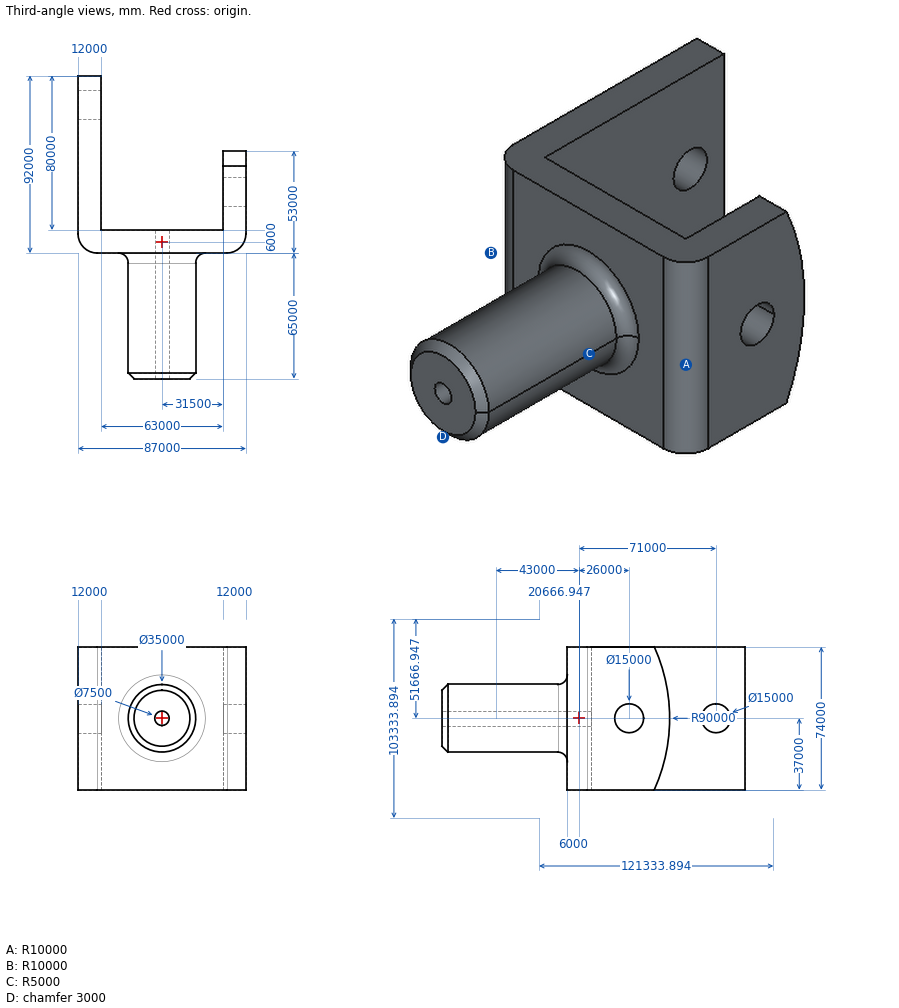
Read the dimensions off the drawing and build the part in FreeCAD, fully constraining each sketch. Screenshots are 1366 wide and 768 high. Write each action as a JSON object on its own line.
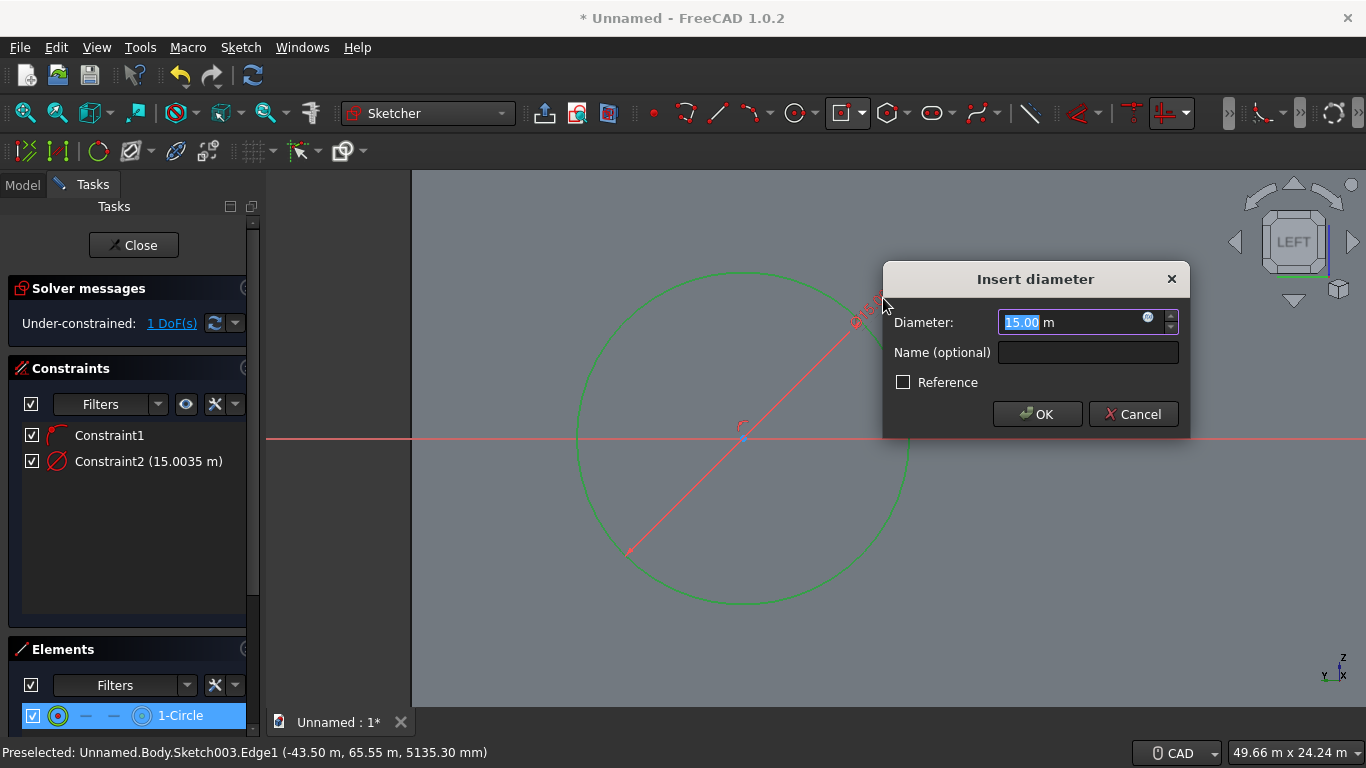
{"action": "key", "text": "ctrl+a"}
{"action": "type", "text": "15000 mm"}
{"action": "key", "text": "Return"}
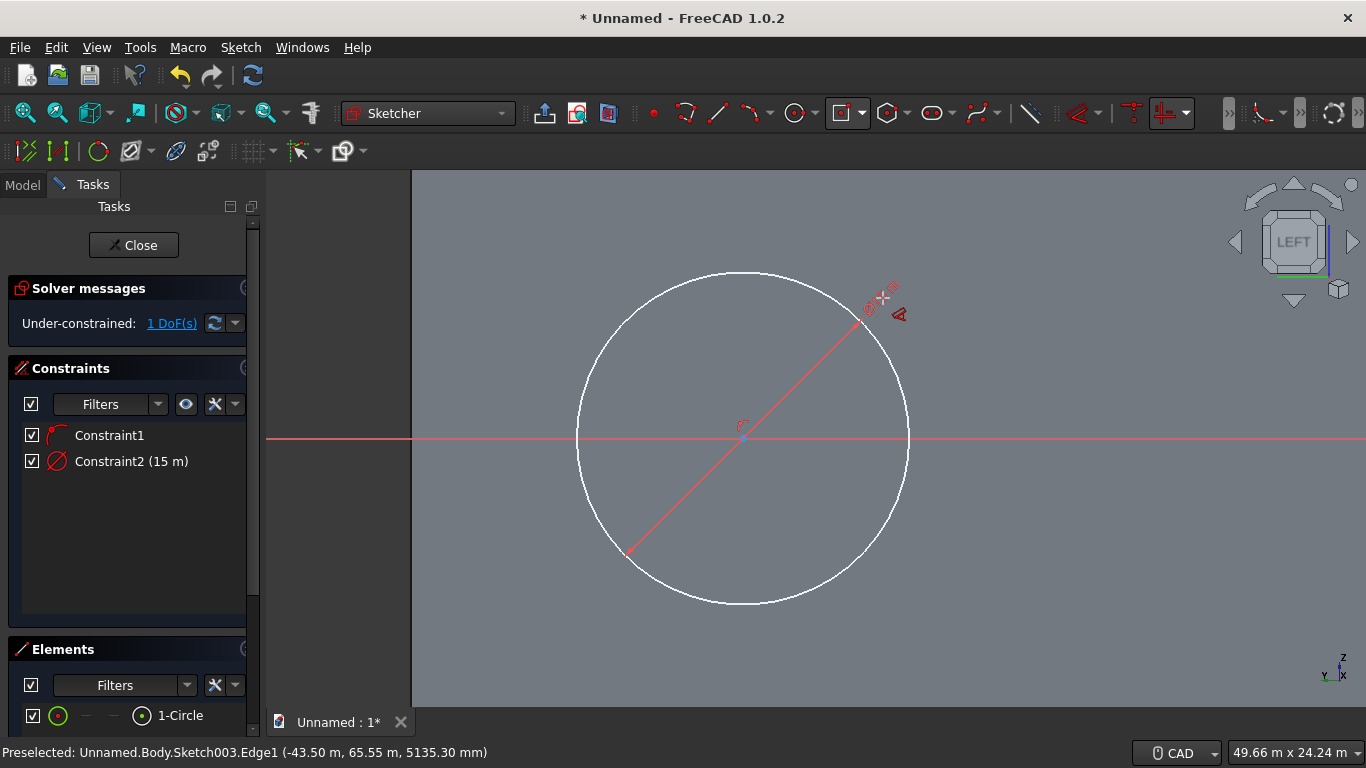
{"action": "left_click", "coordinate": [743, 438]}
{"action": "left_click", "coordinate": [972, 472]}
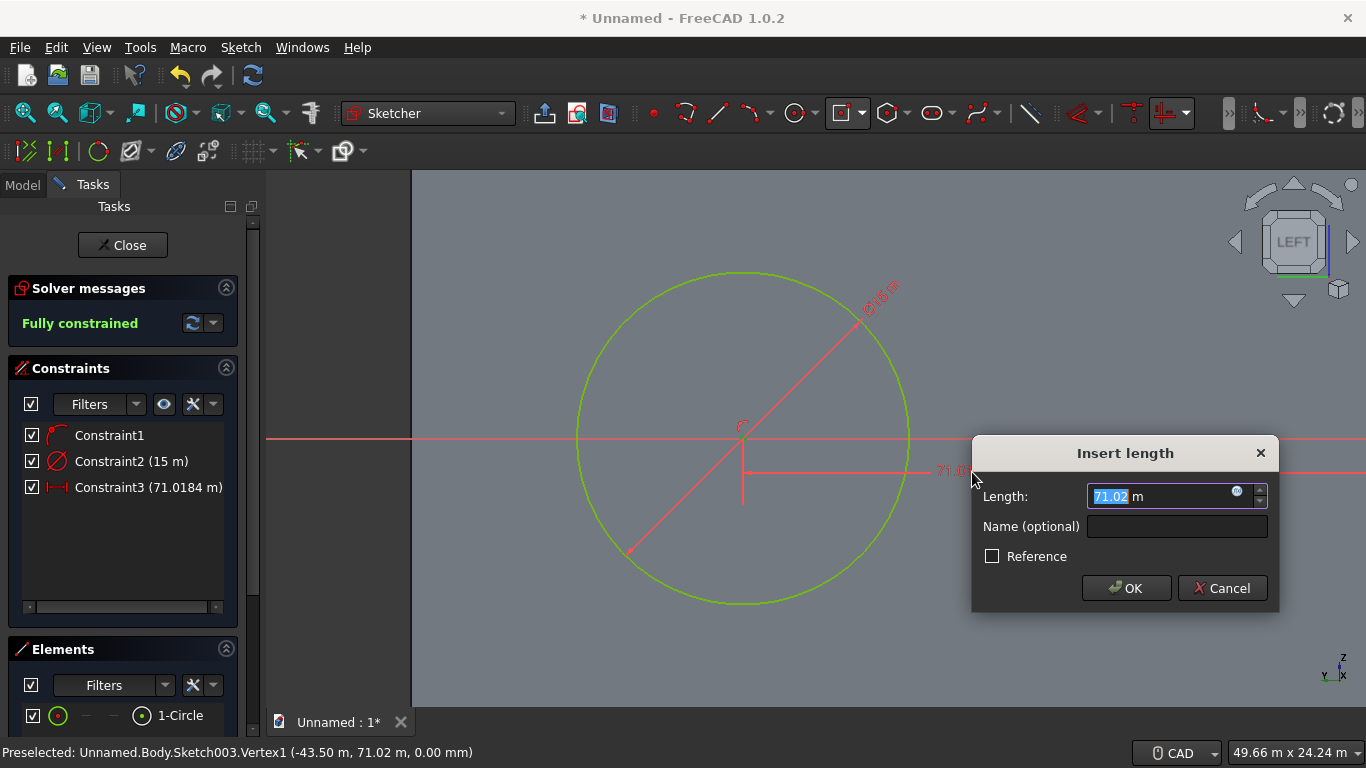
{"action": "key", "text": "ctrl+a"}
{"action": "type", "text": "71000 mm"}
{"action": "key", "text": "Return"}
{"action": "key", "text": "Escape"}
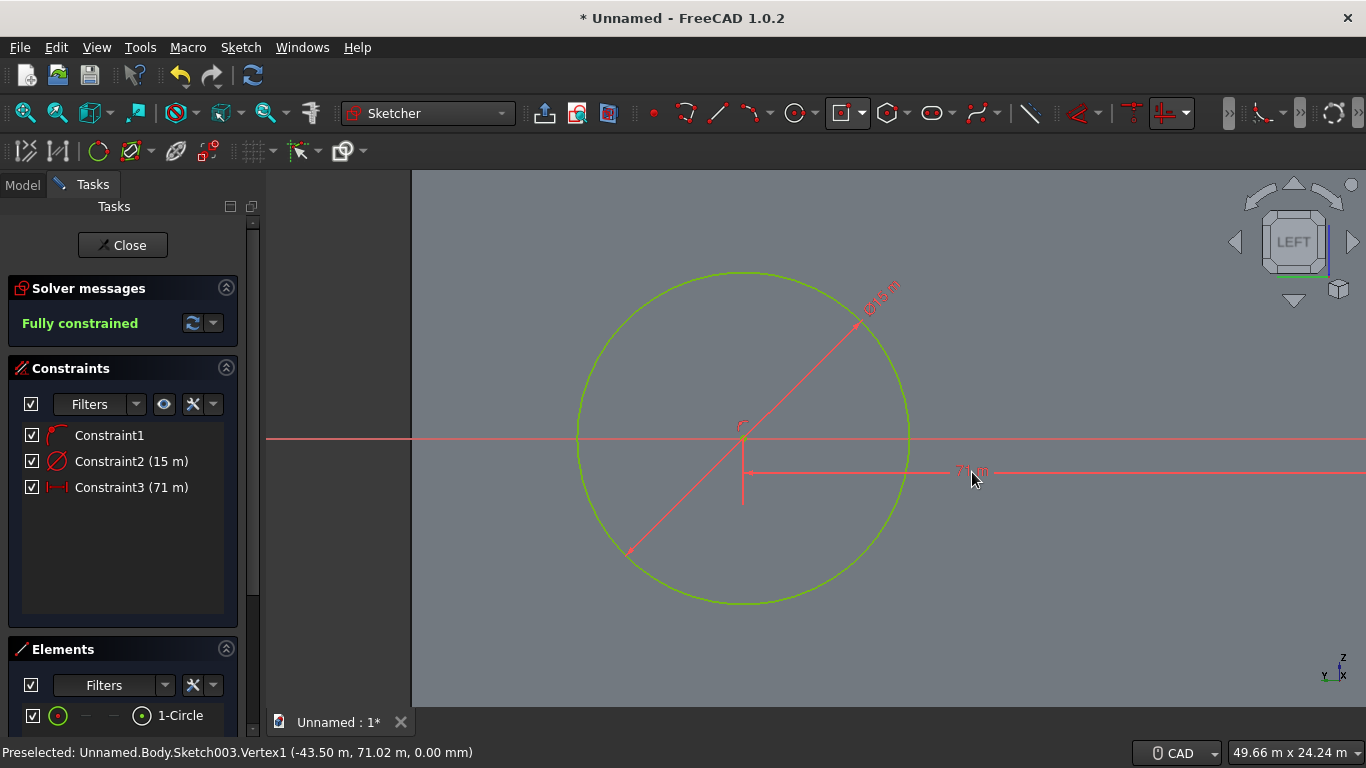
{"action": "left_click", "coordinate": [123, 245]}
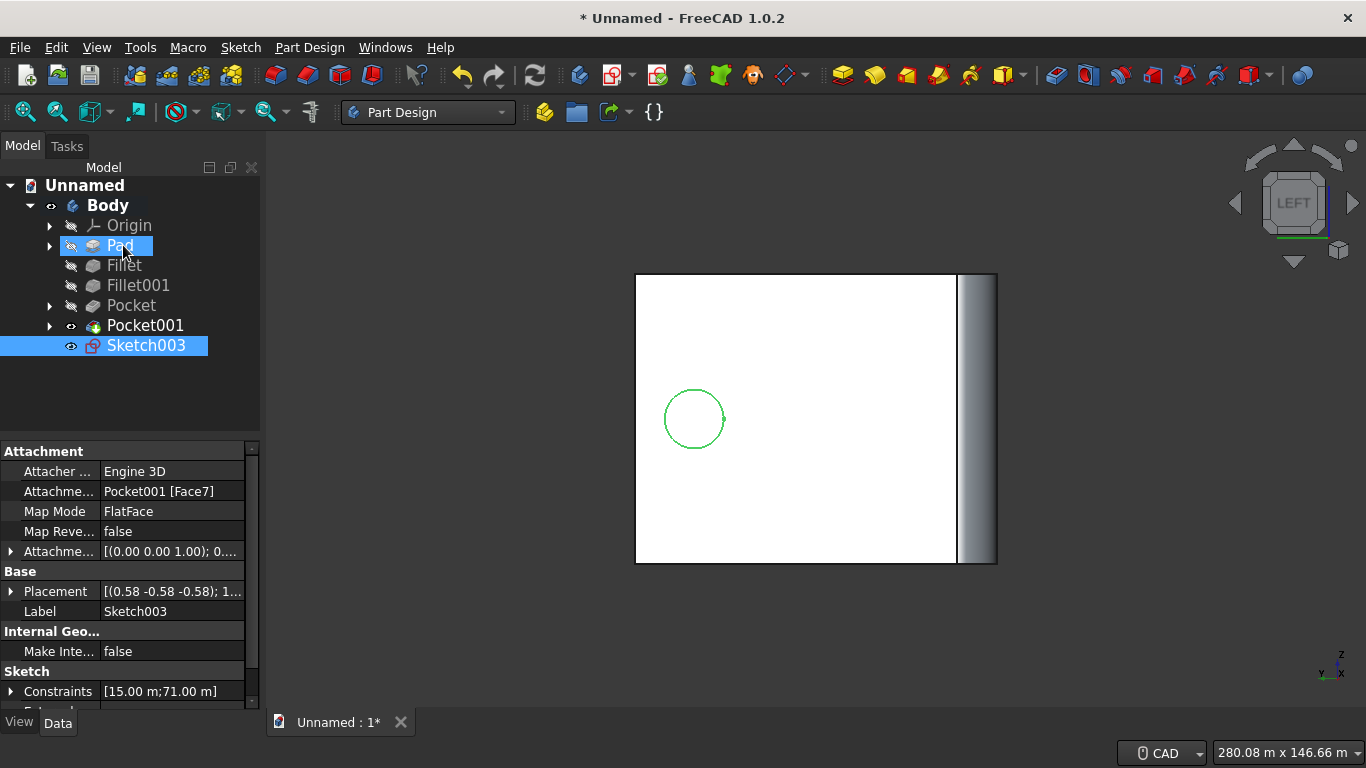
{"action": "left_click", "coordinate": [1058, 76]}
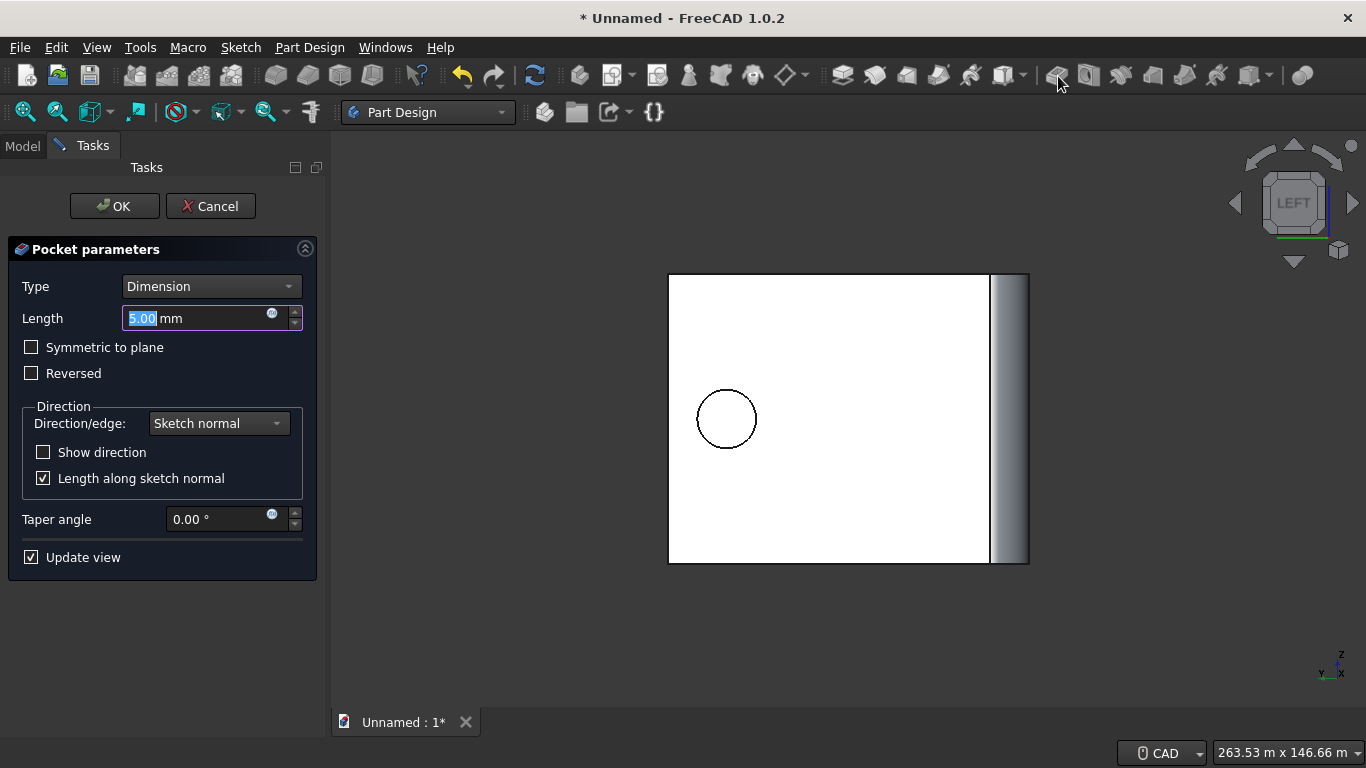
{"action": "type", "text": "12000"}
{"action": "key", "text": "Tab"}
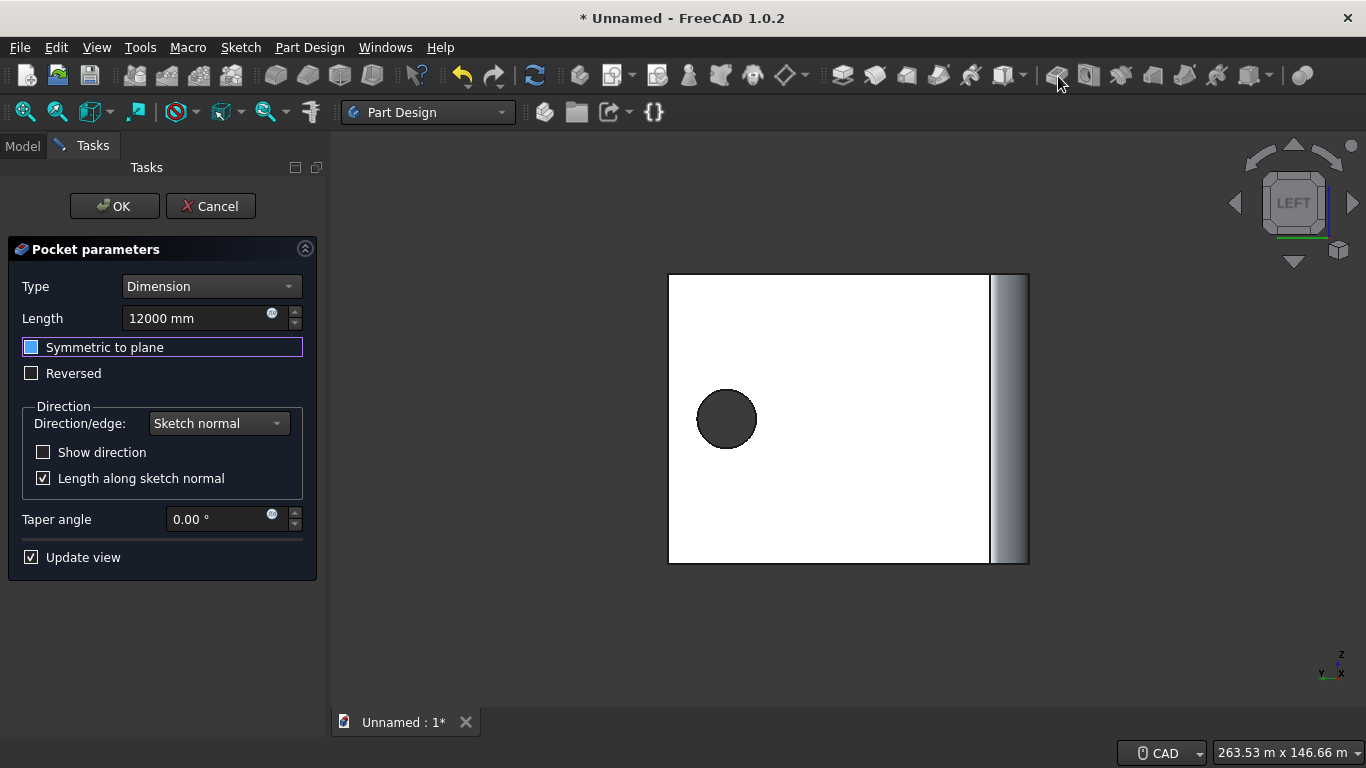
{"action": "left_click", "coordinate": [115, 206]}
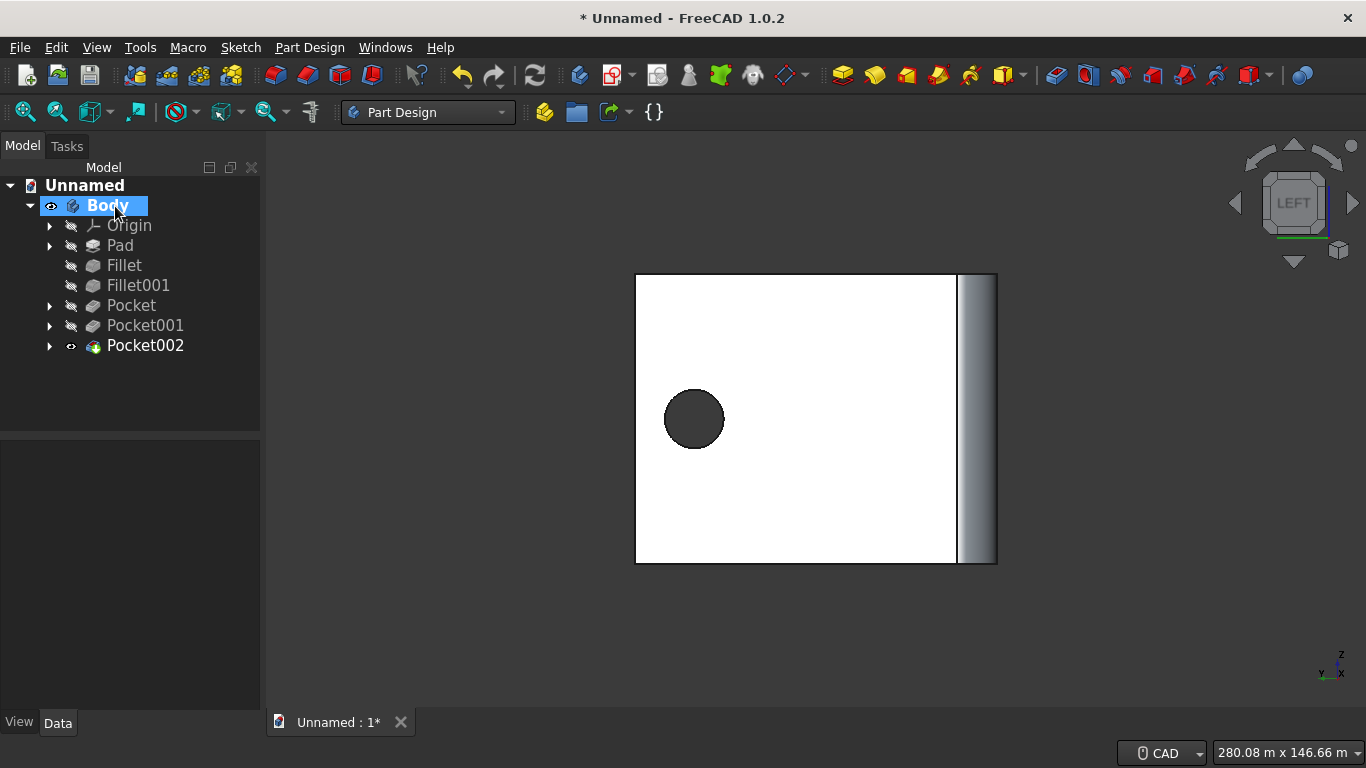
{"action": "key", "text": "0"}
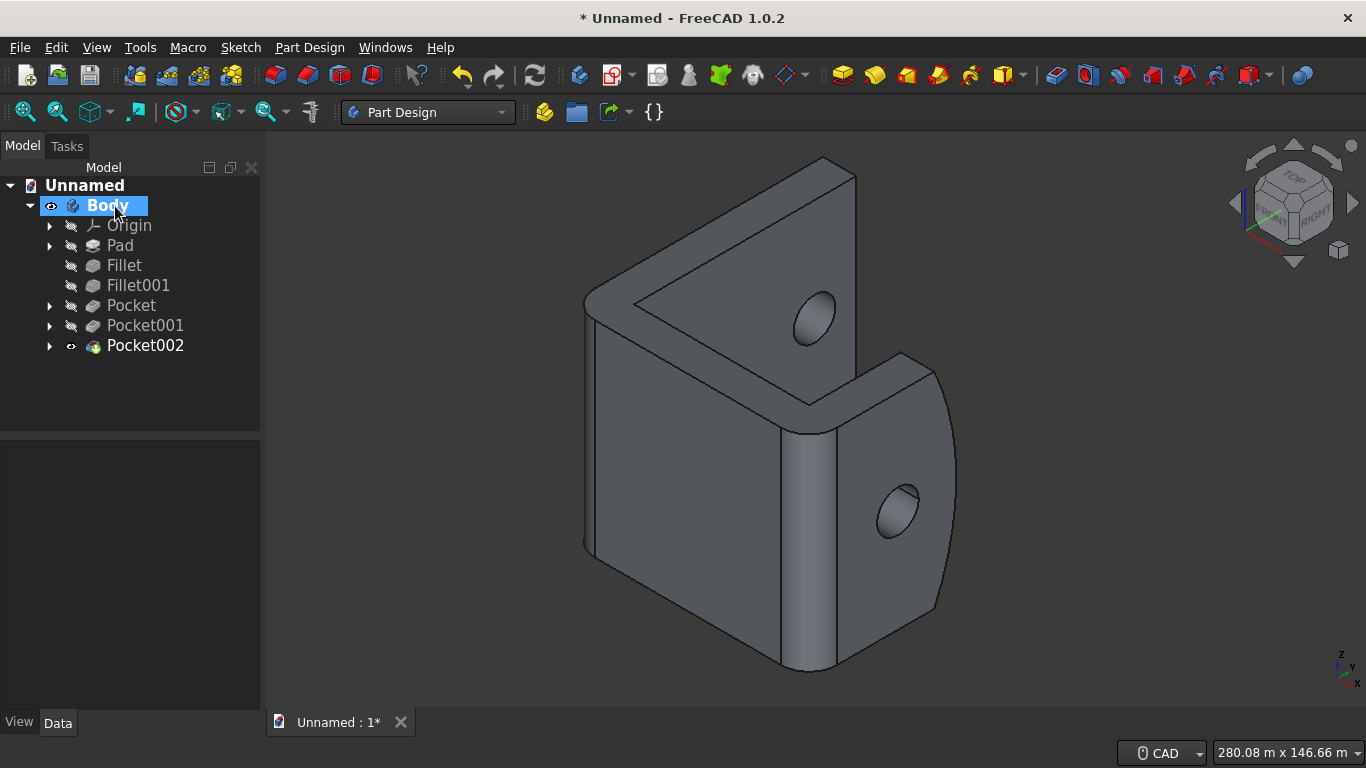
{"action": "left_click", "coordinate": [688, 492]}